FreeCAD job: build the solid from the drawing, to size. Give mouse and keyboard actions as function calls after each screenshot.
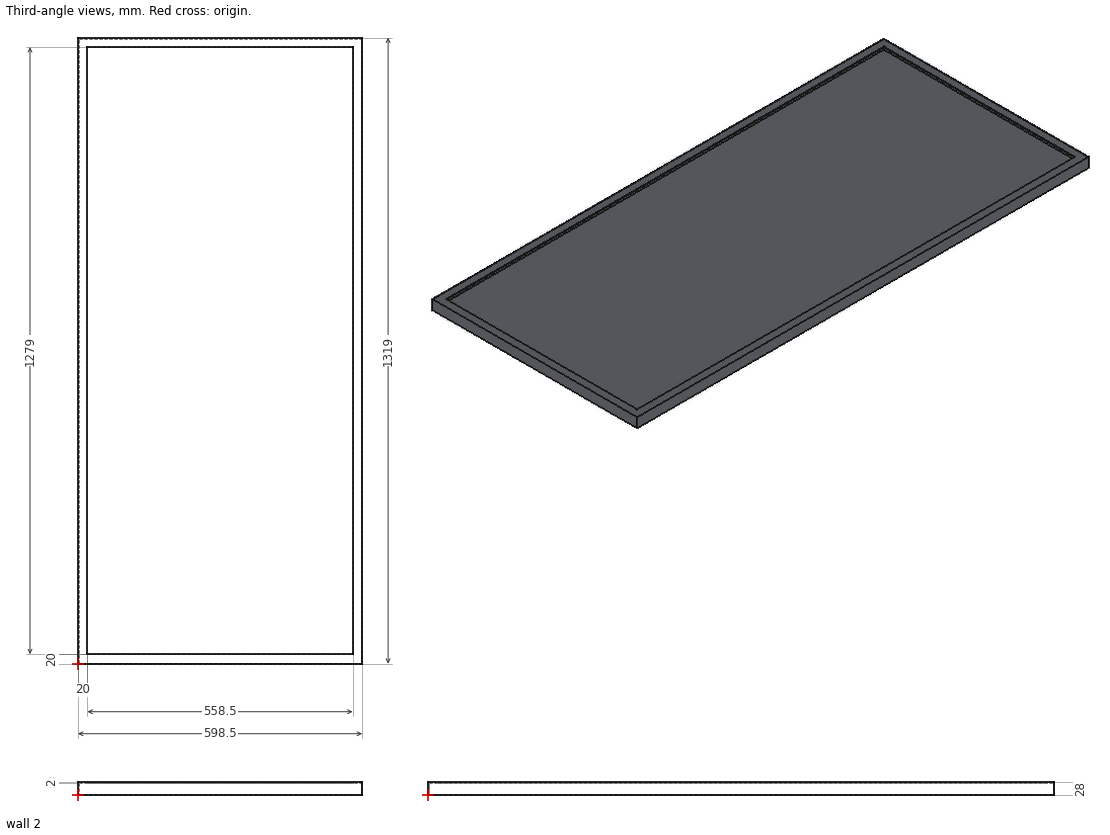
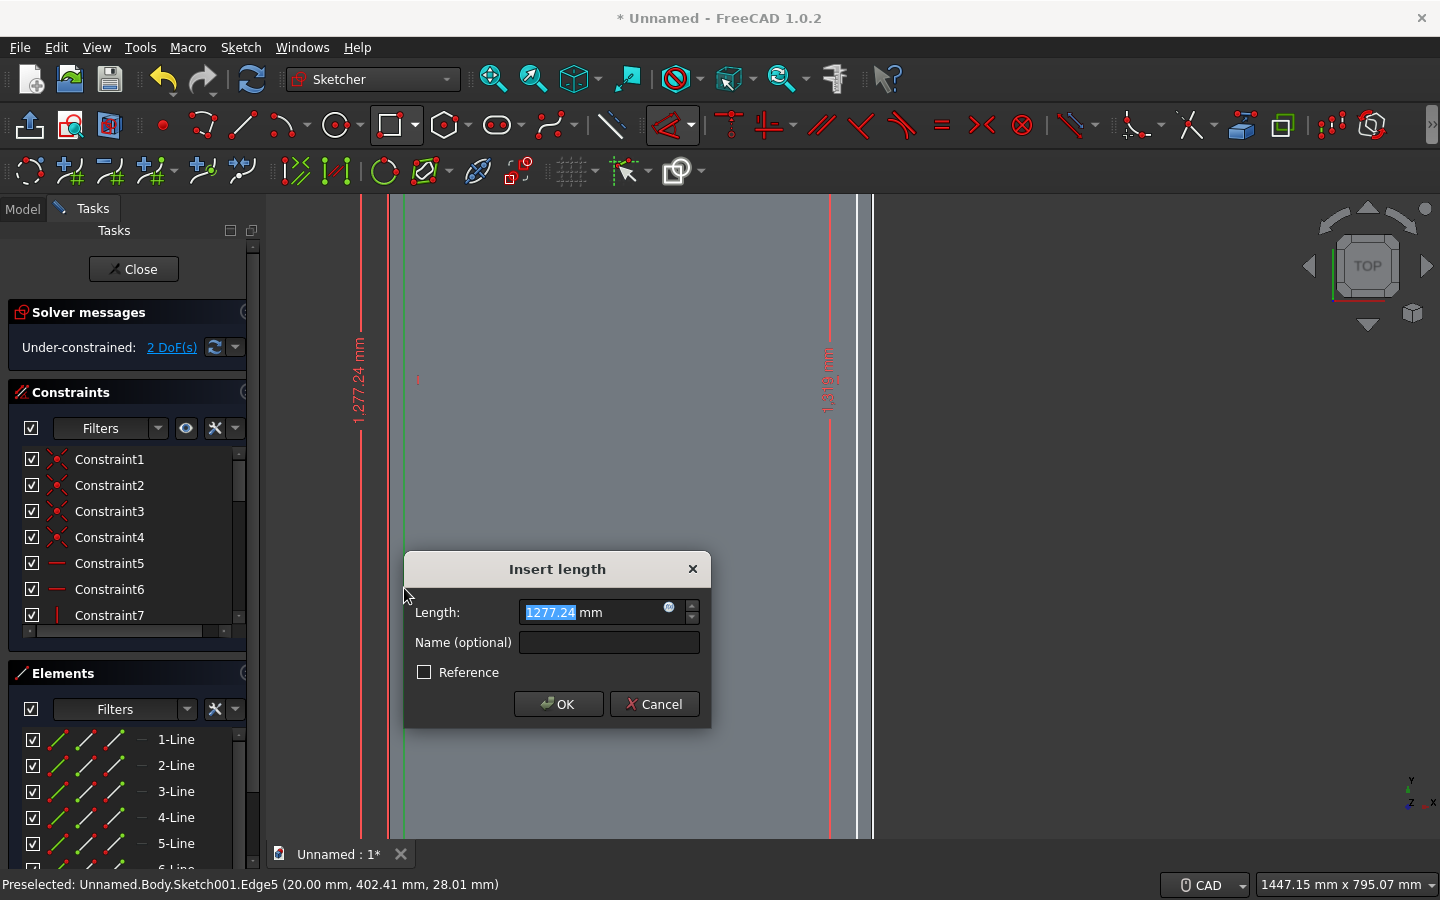
text(1279)
key(Return)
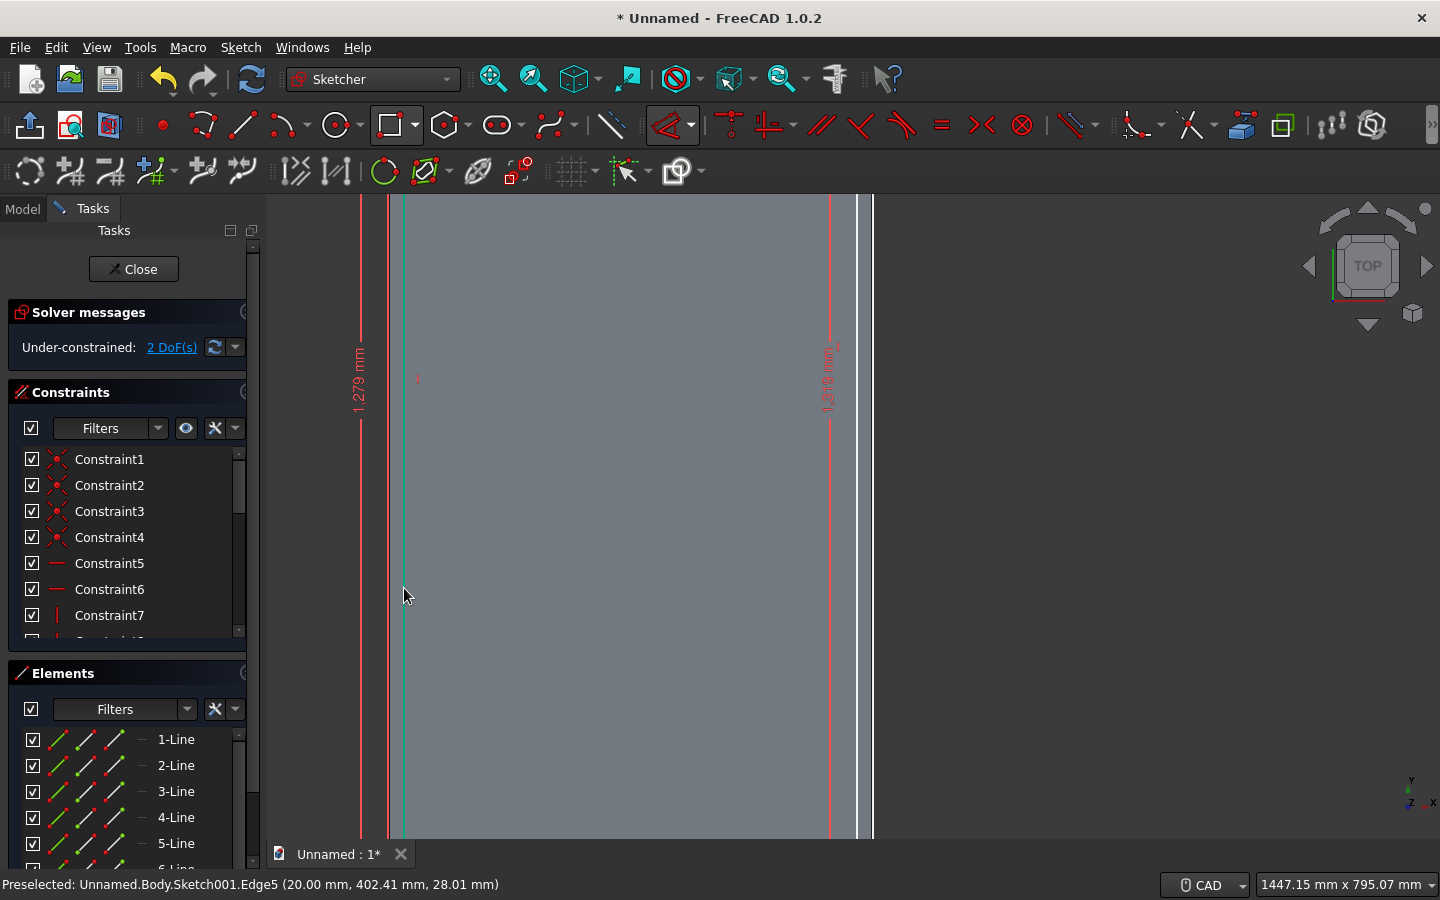
scroll(874, 596, down, 5)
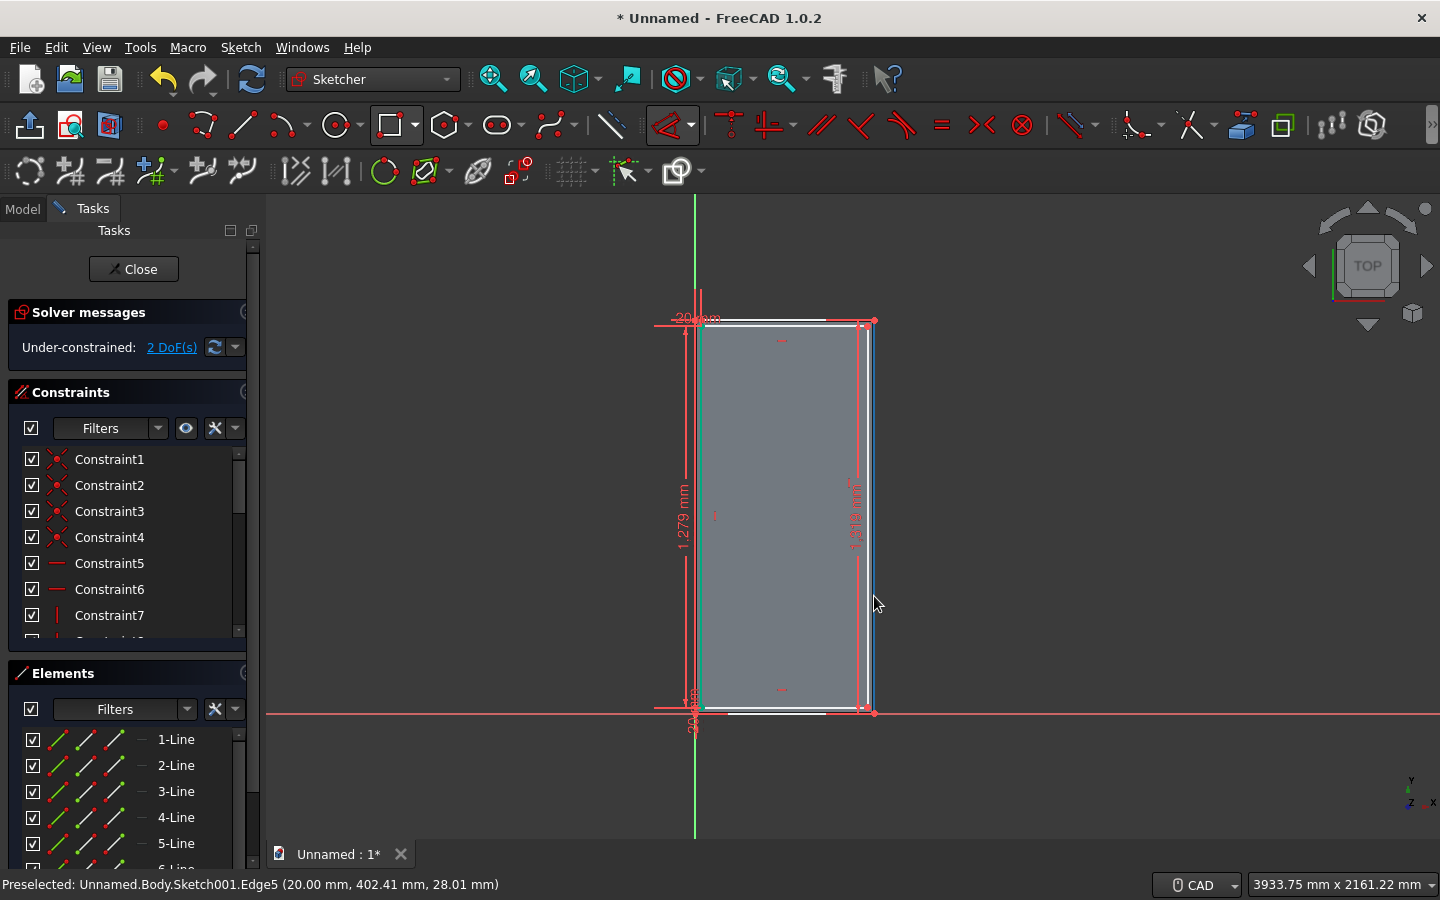
scroll(749, 714, up, 5)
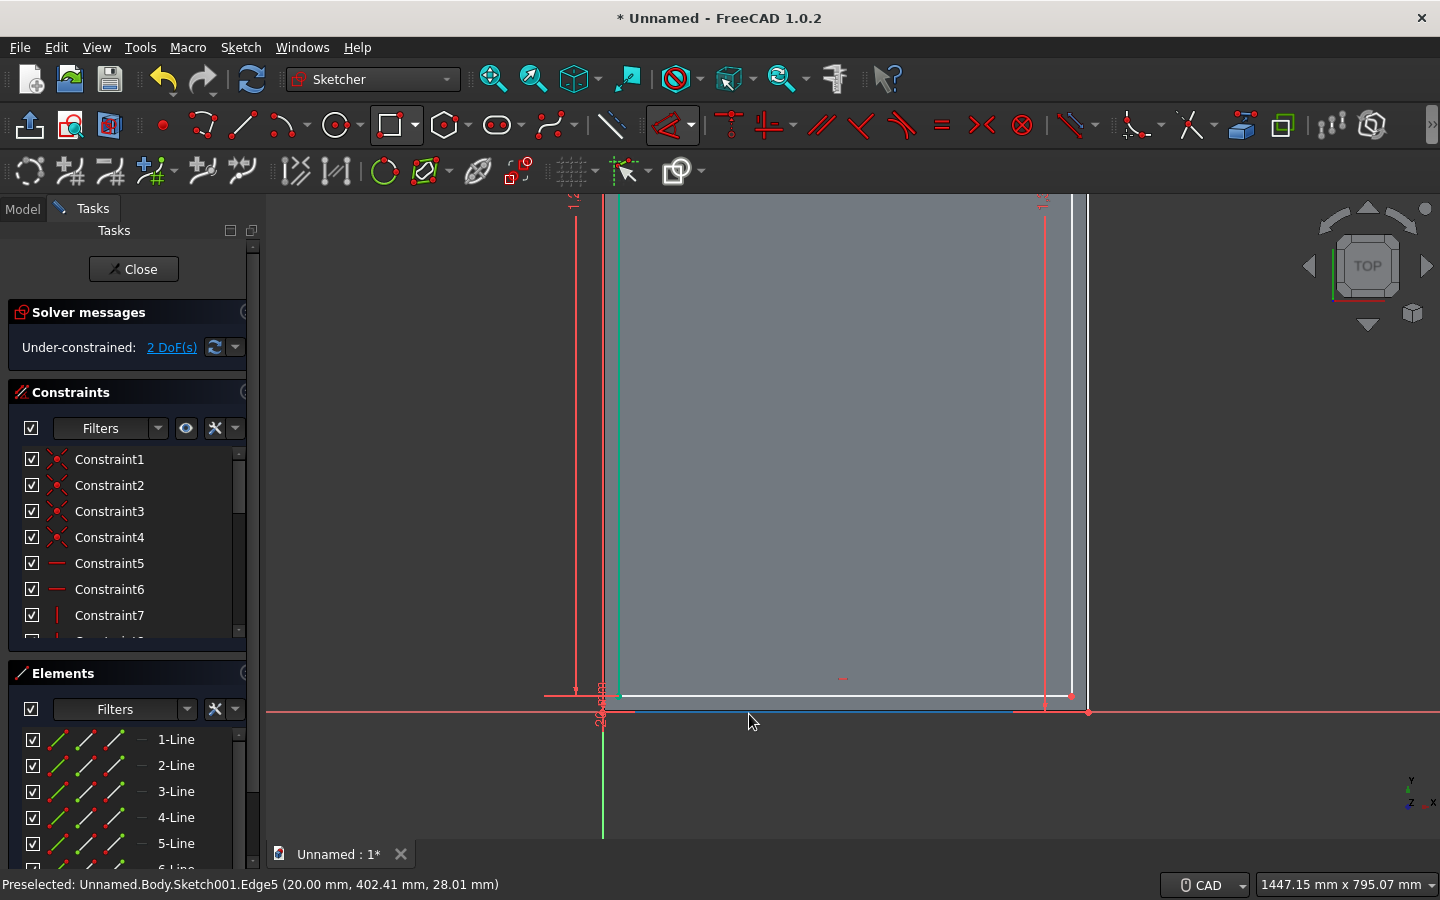
click(748, 712)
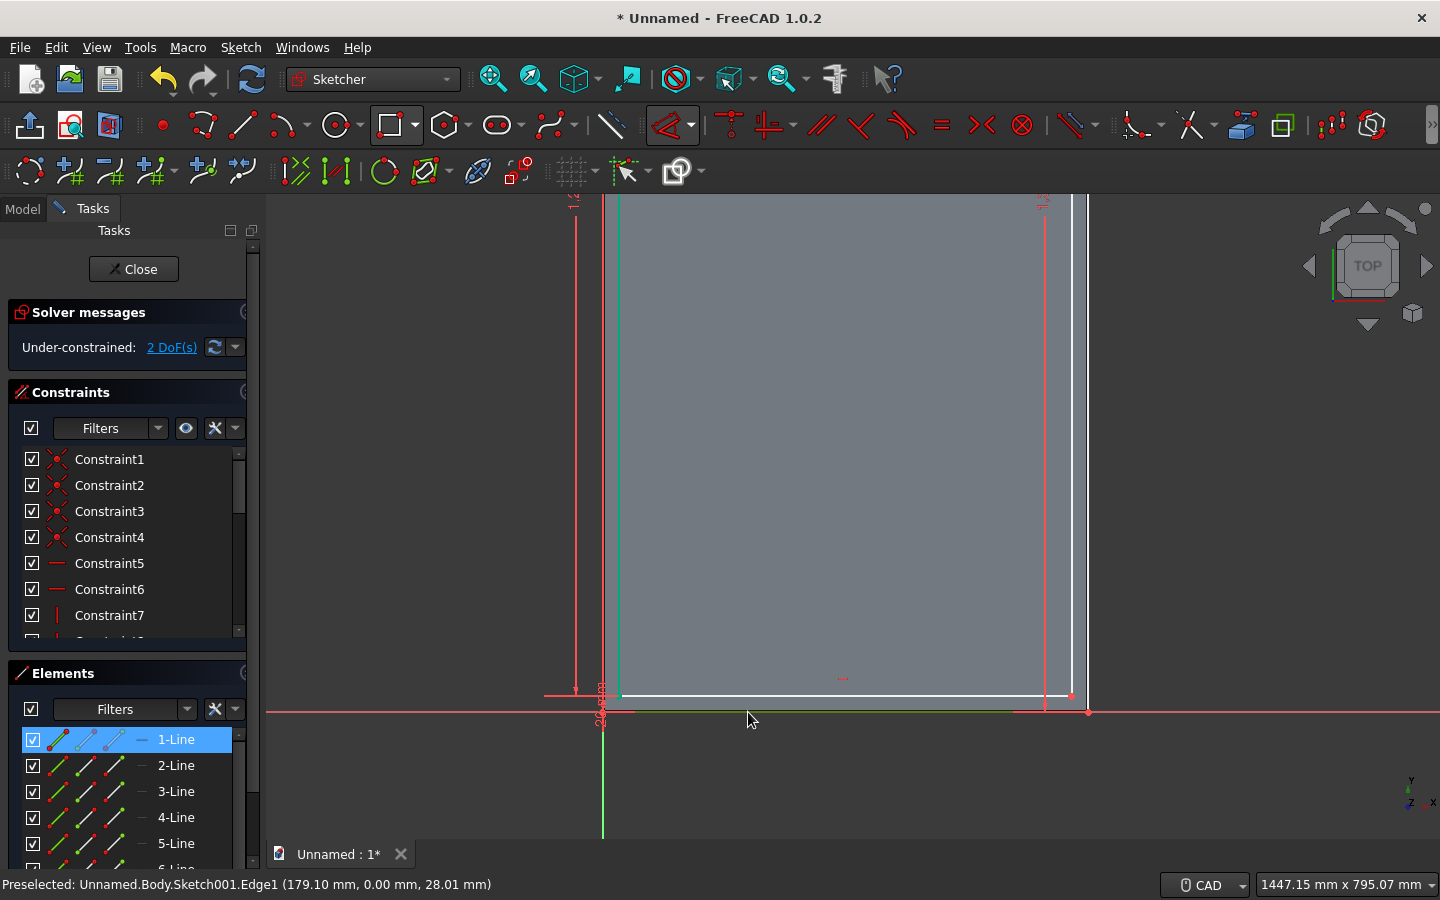
key(l)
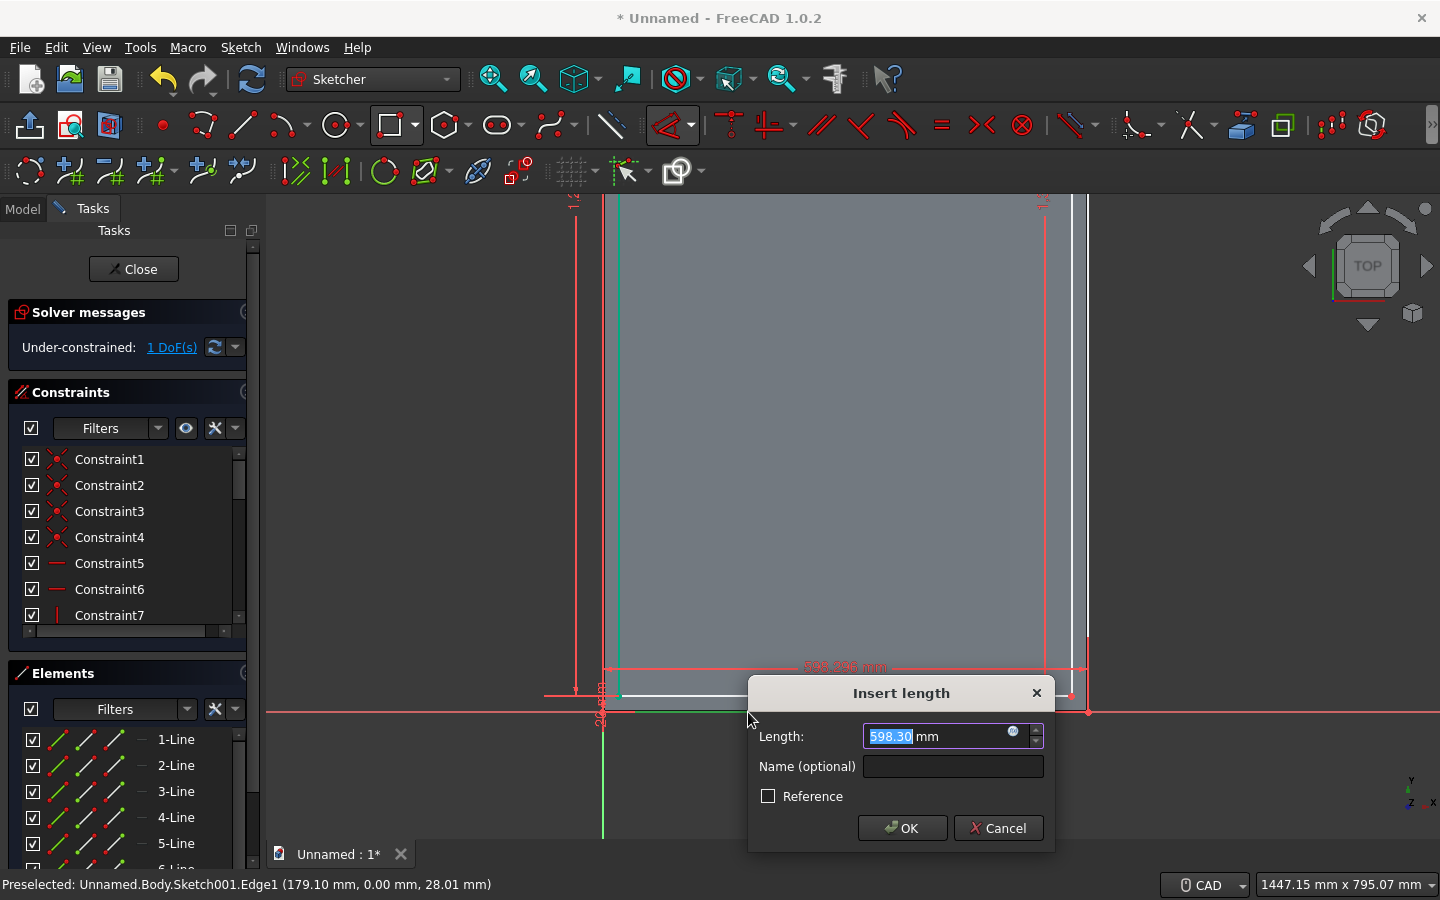
text(598.5)
key(Return)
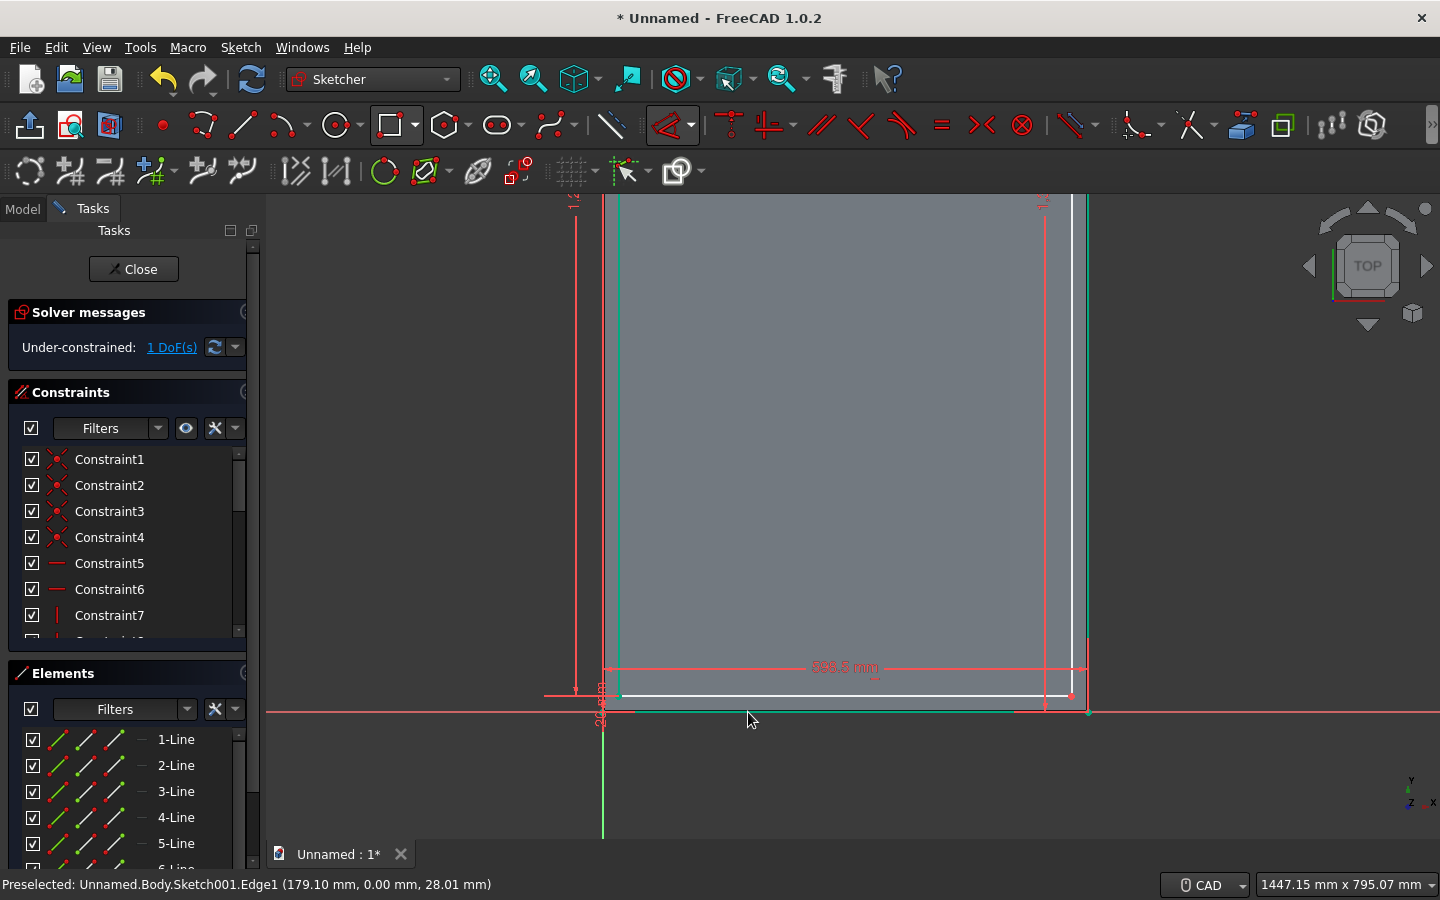
click(755, 696)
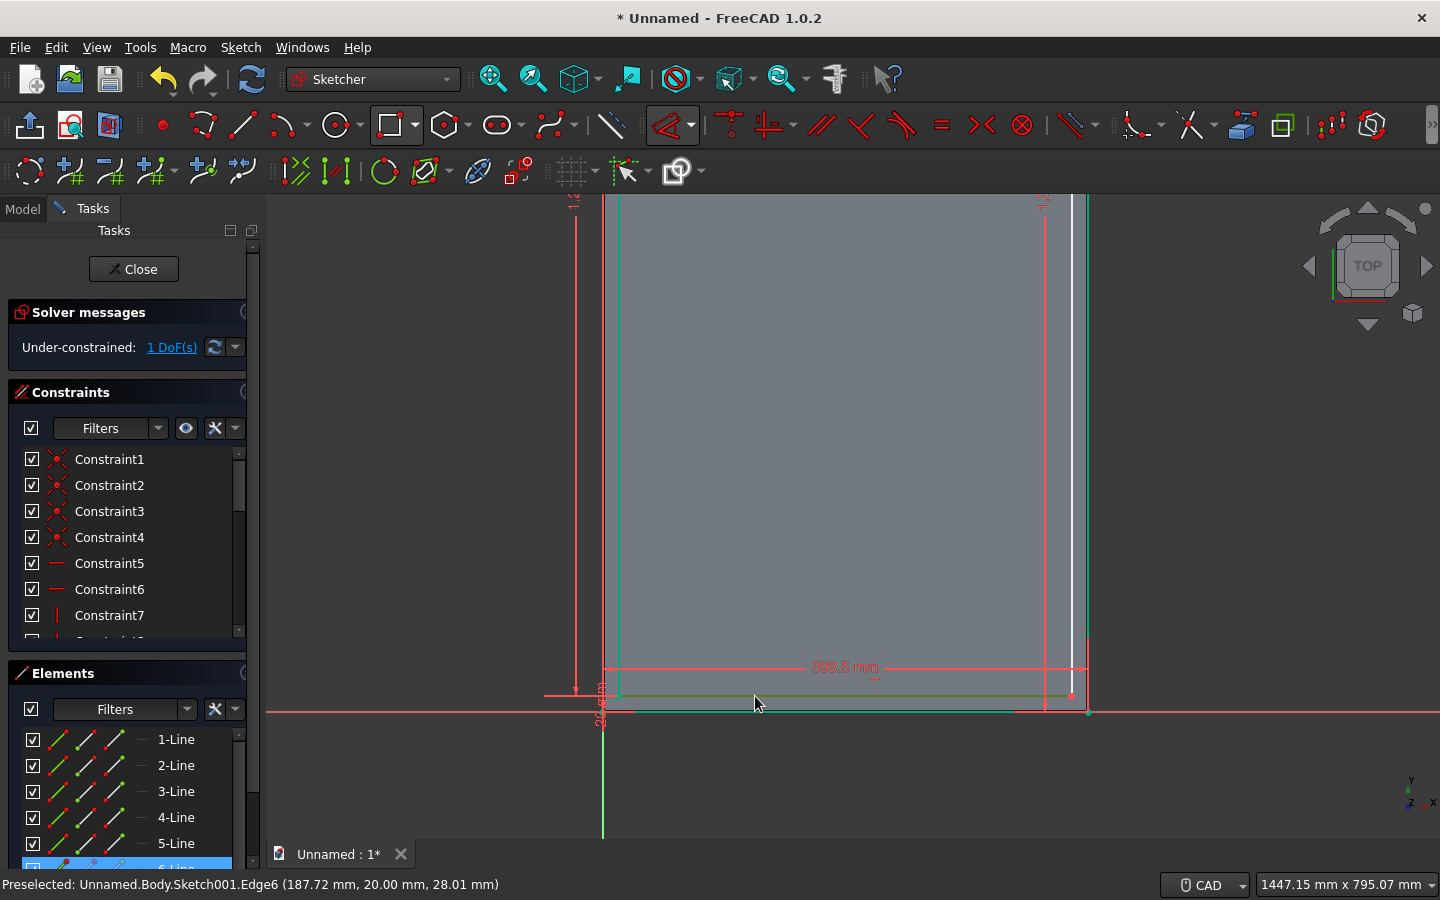
key(l)